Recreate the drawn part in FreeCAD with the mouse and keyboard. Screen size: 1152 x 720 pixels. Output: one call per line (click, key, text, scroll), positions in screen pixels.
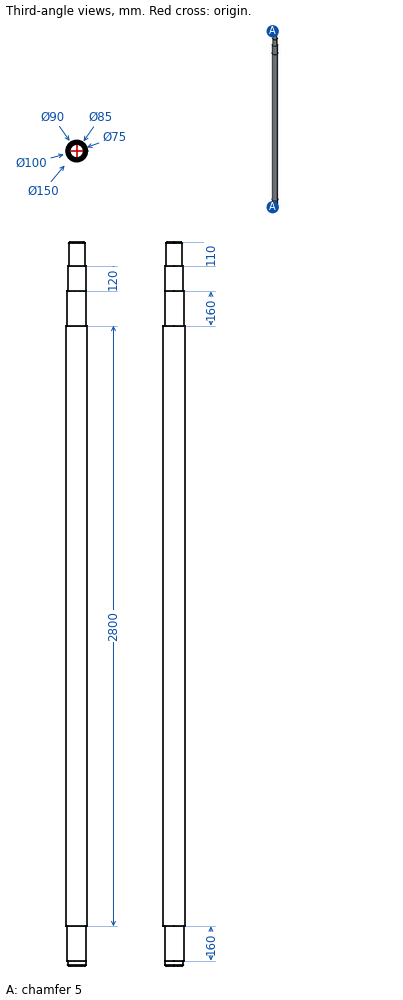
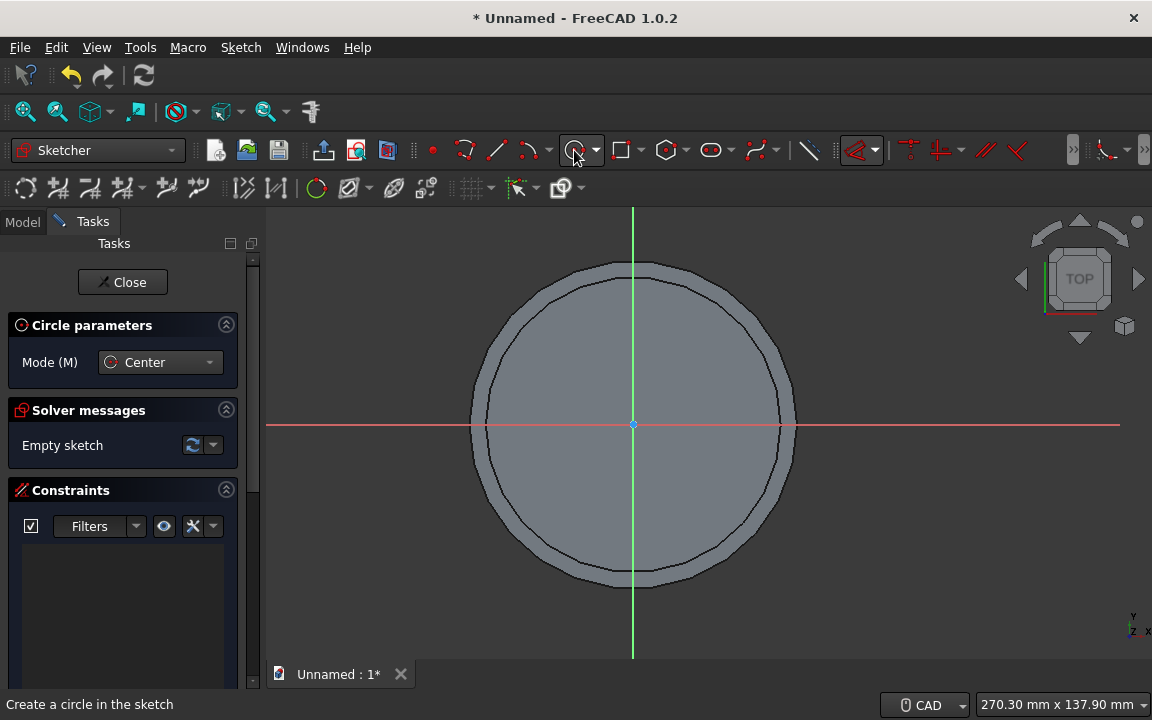
click(633, 425)
click(732, 326)
key(Escape)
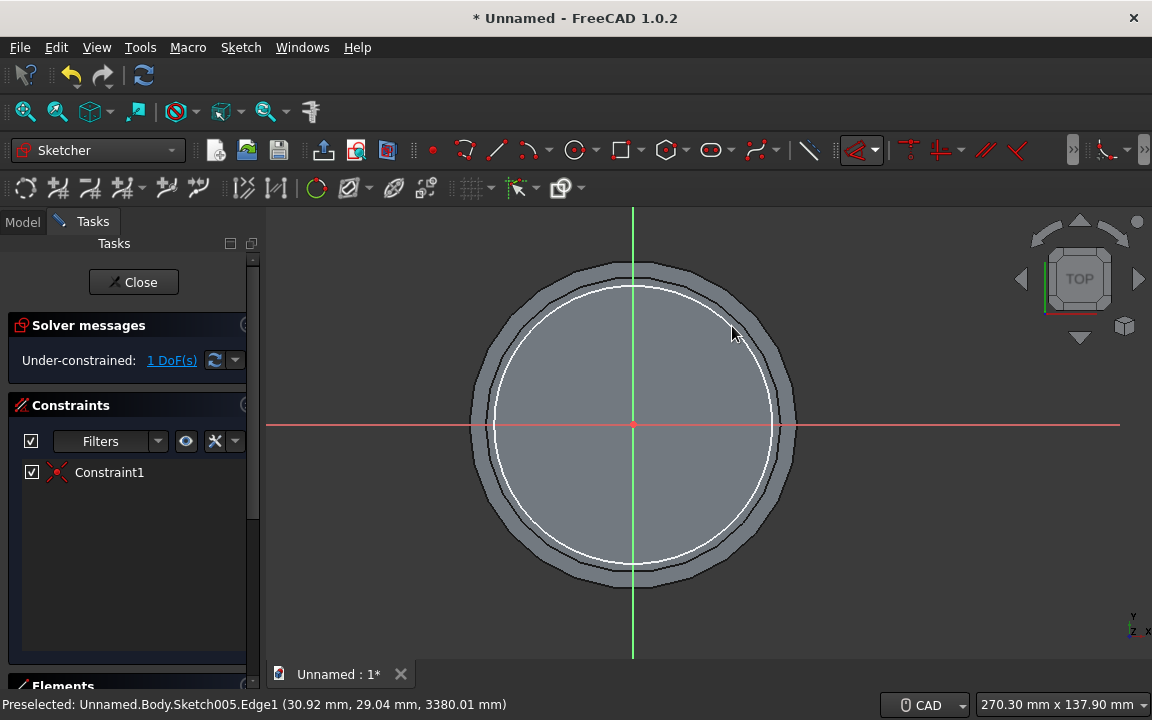
click(731, 326)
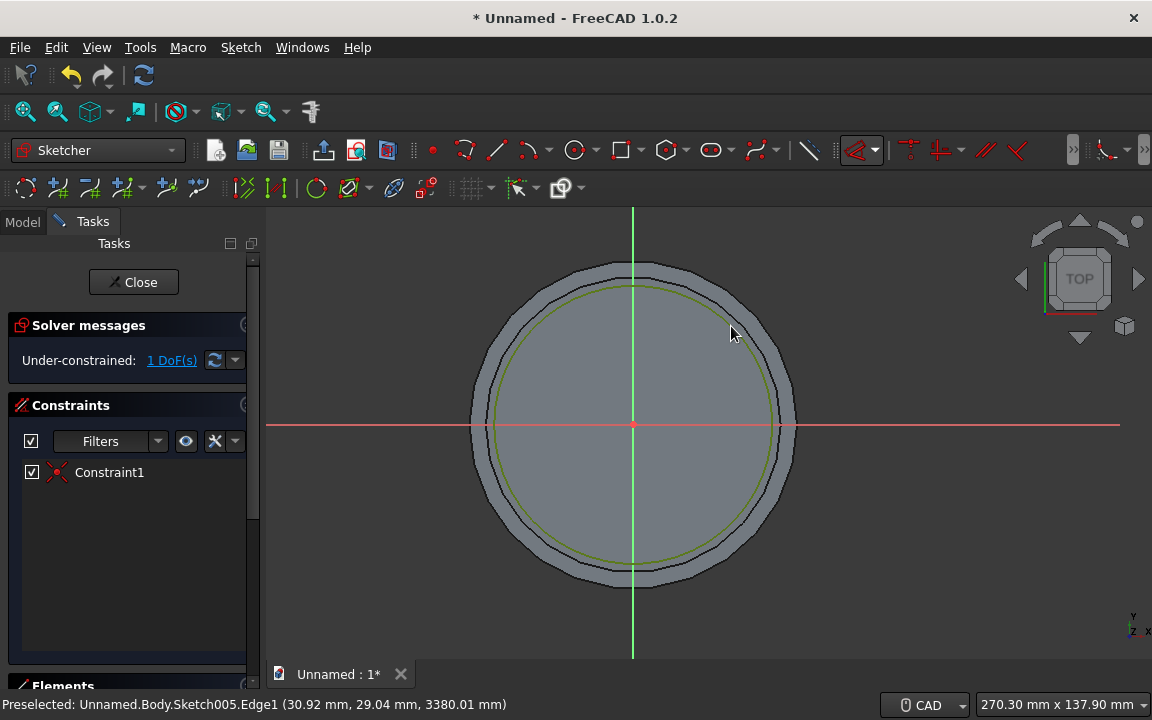
click(878, 150)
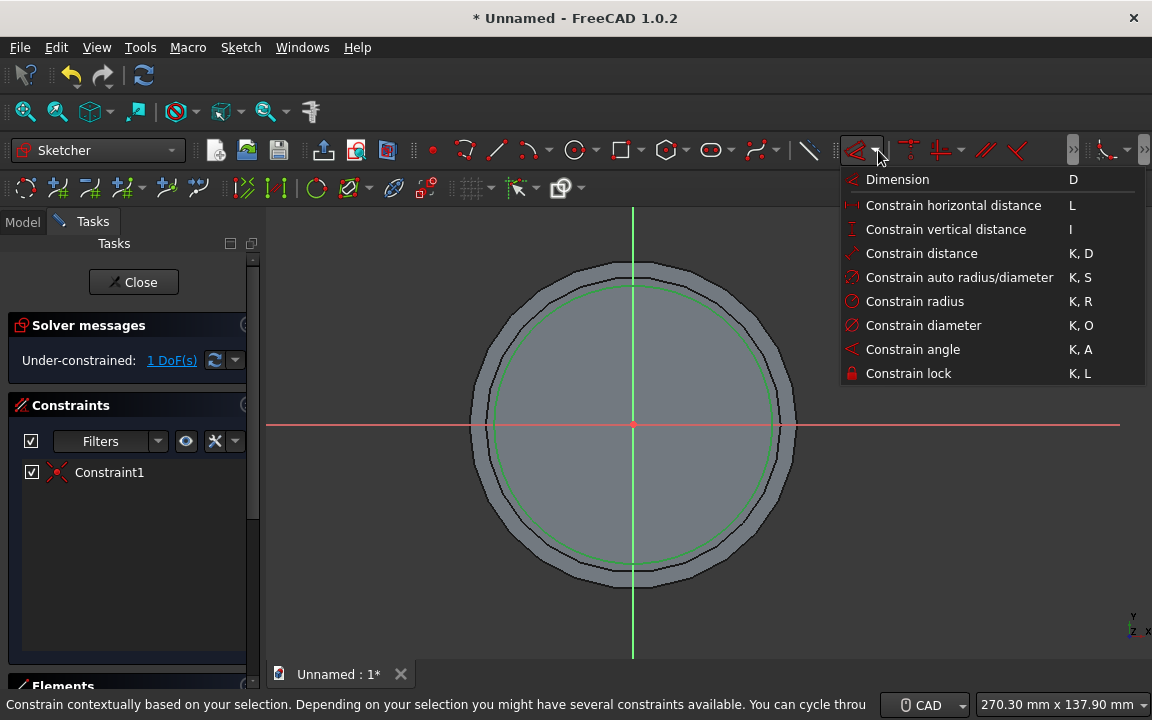
click(993, 325)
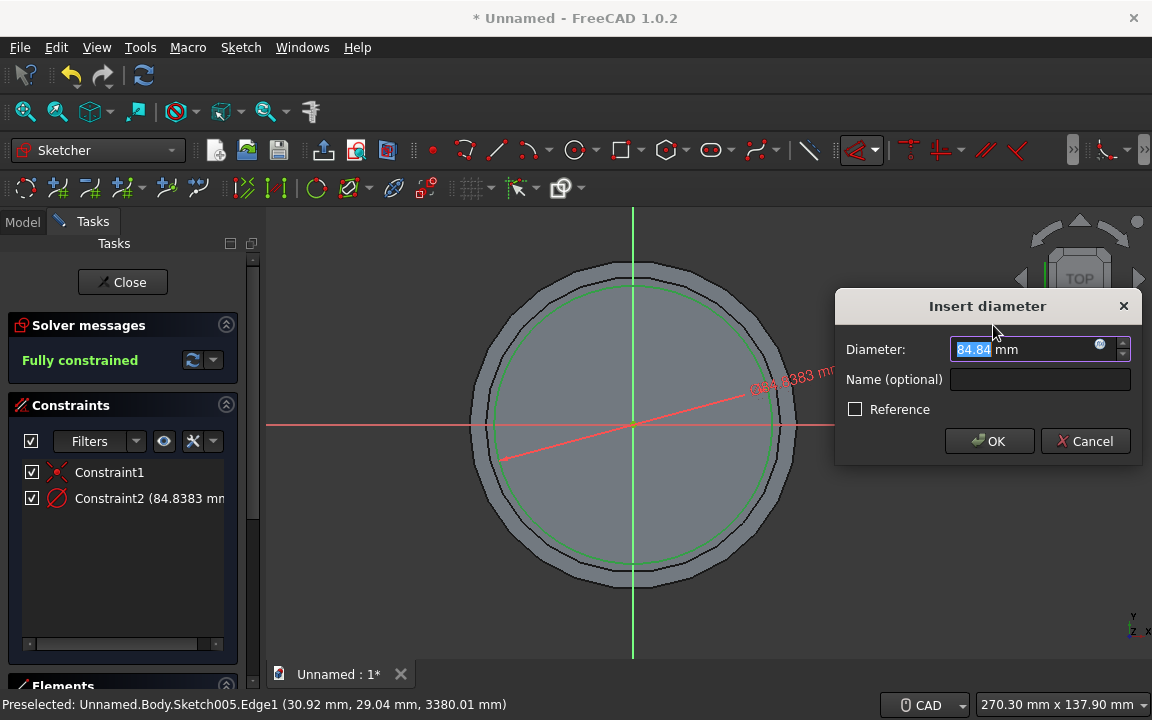
text(85)
key(Return)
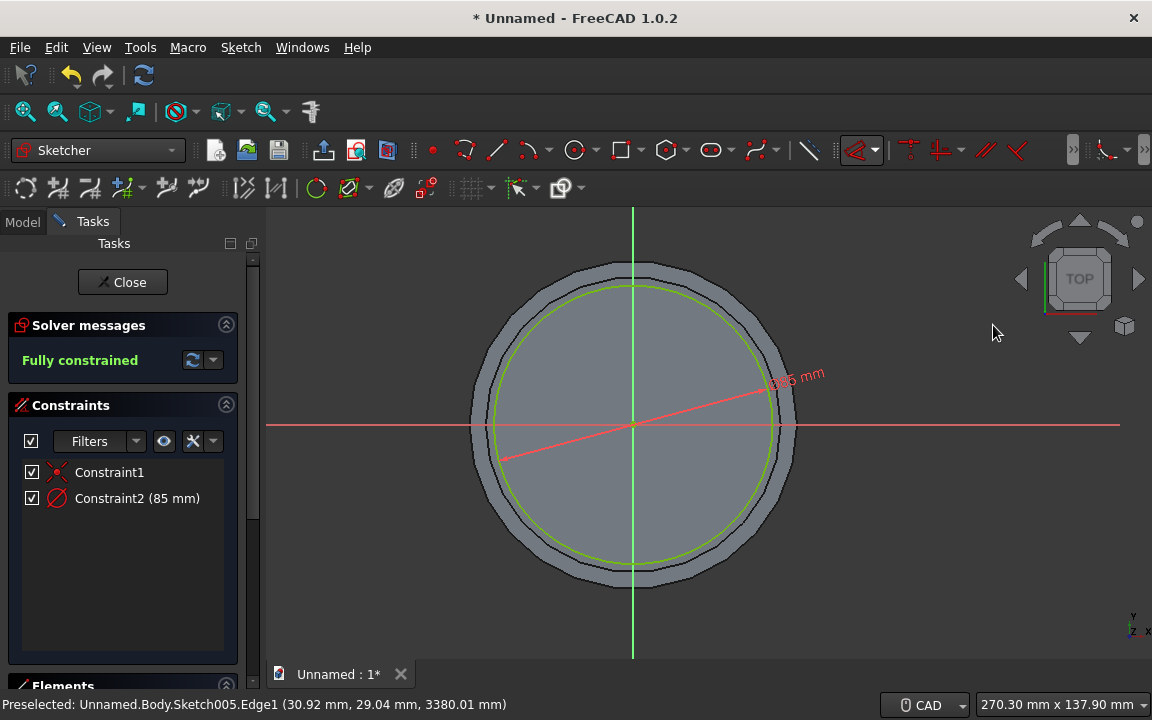
click(123, 282)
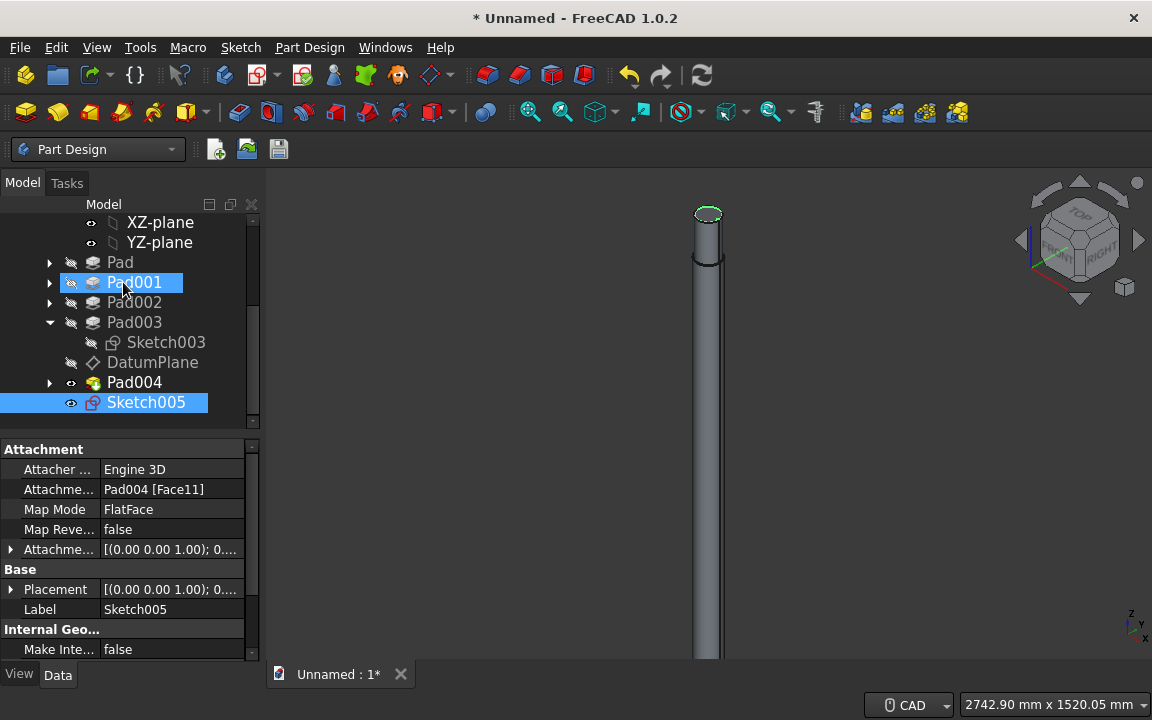
click(26, 112)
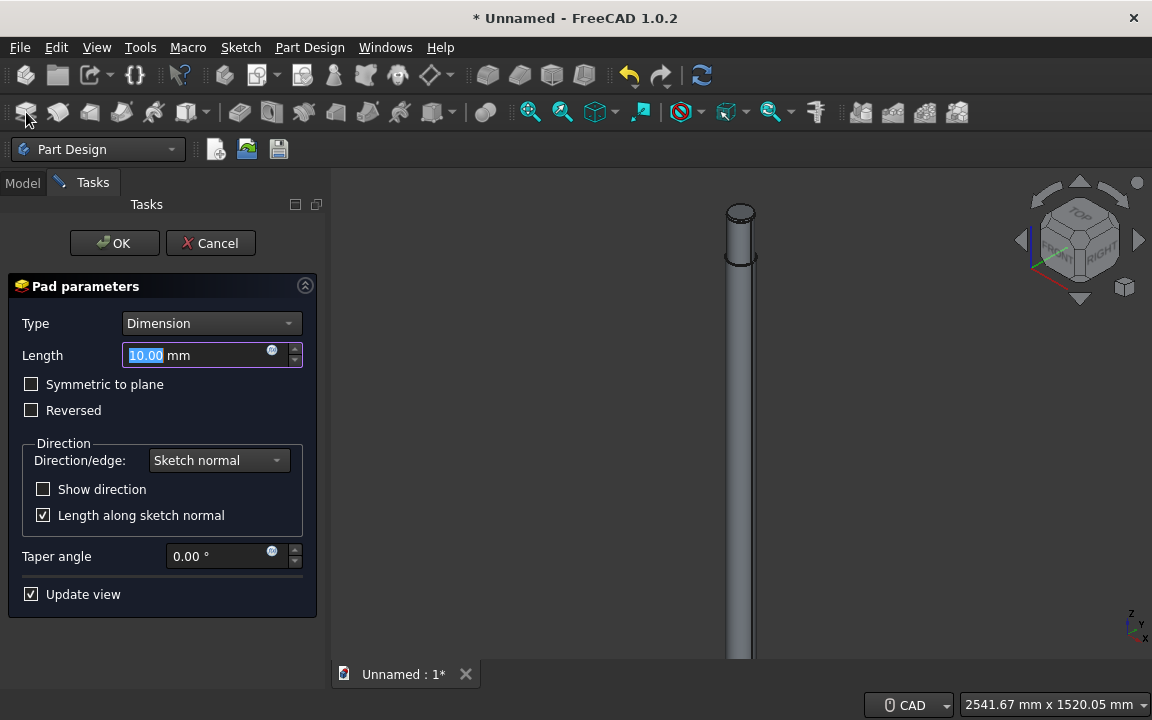
text(120)
key(Tab)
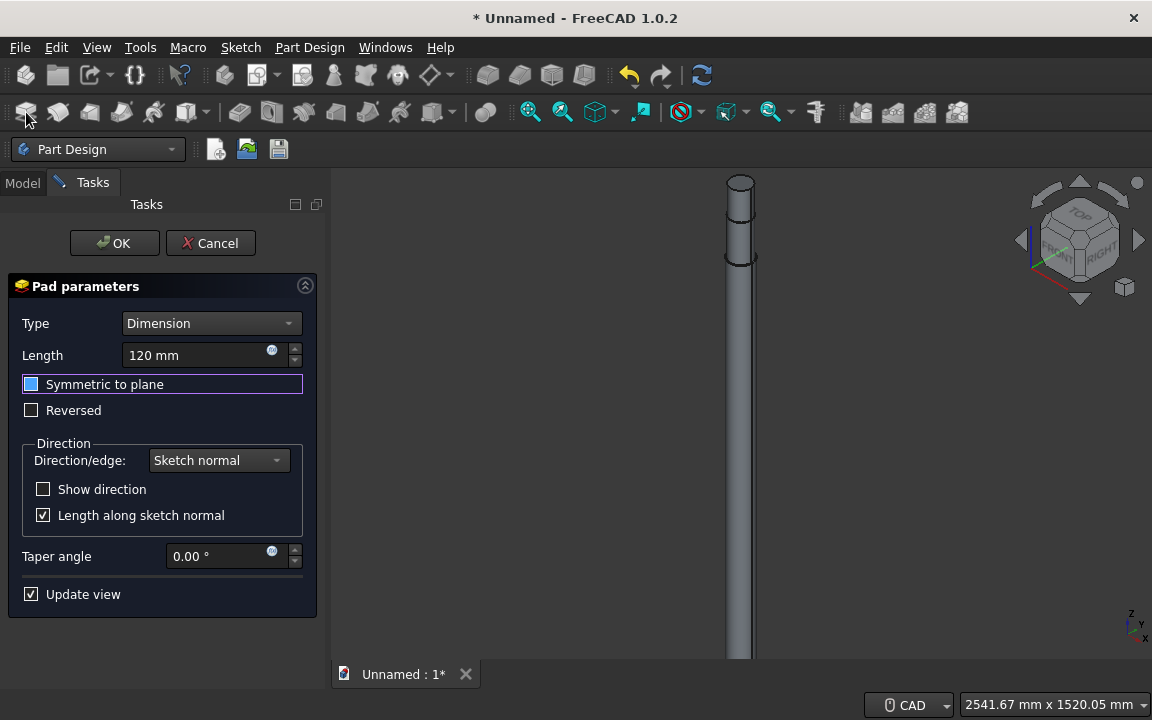
click(115, 243)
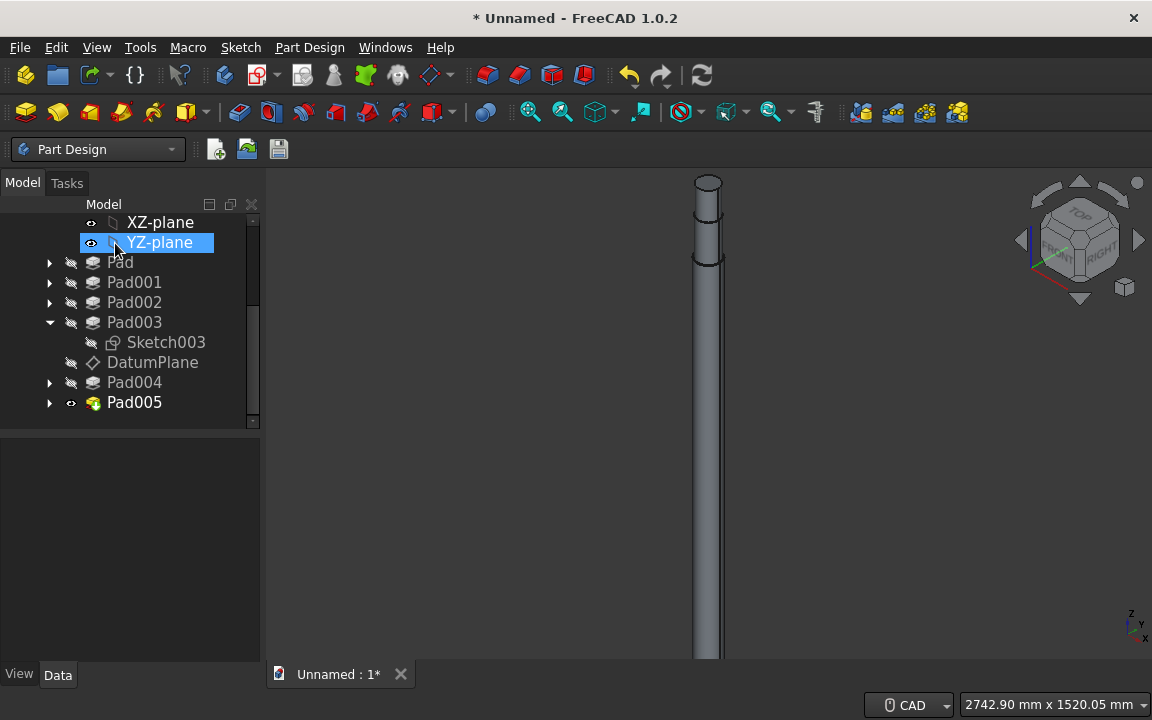
click(532, 112)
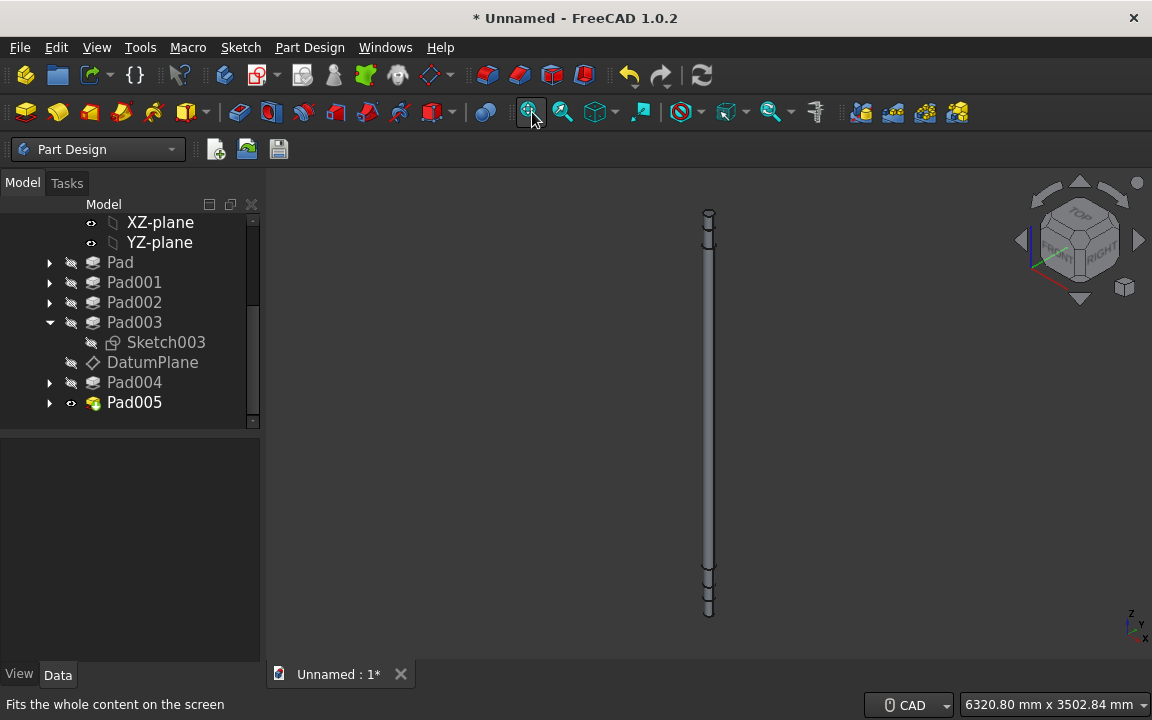
scroll(709, 212, up, 4)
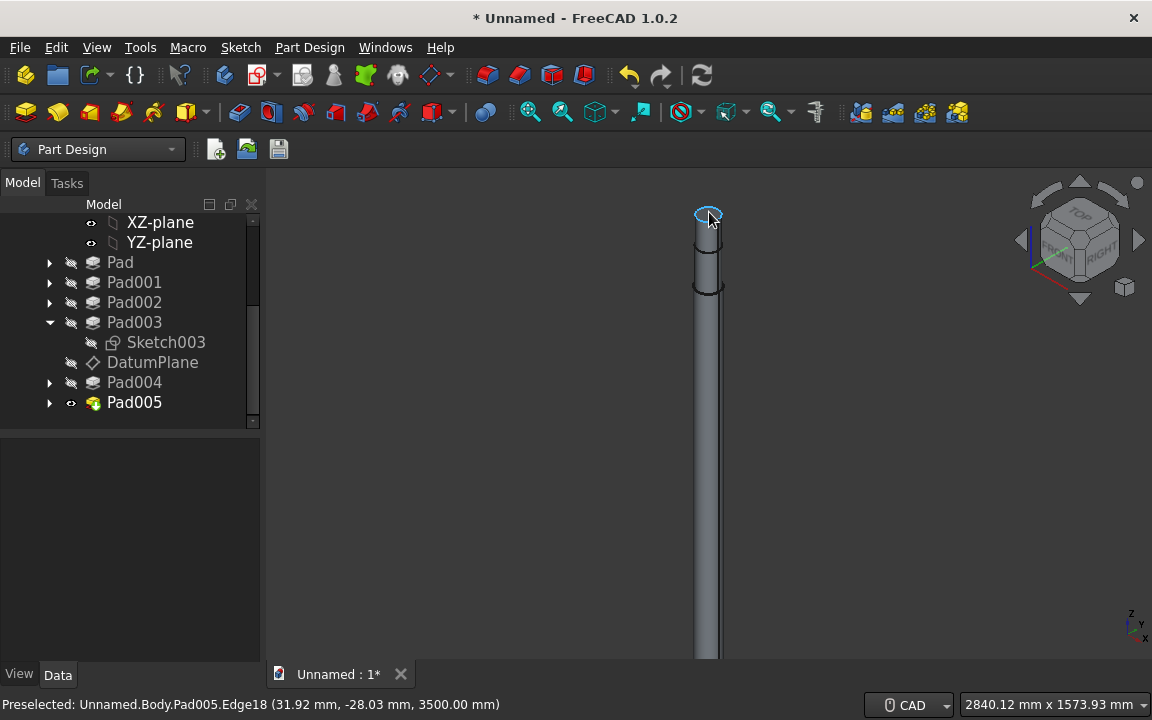
click(711, 212)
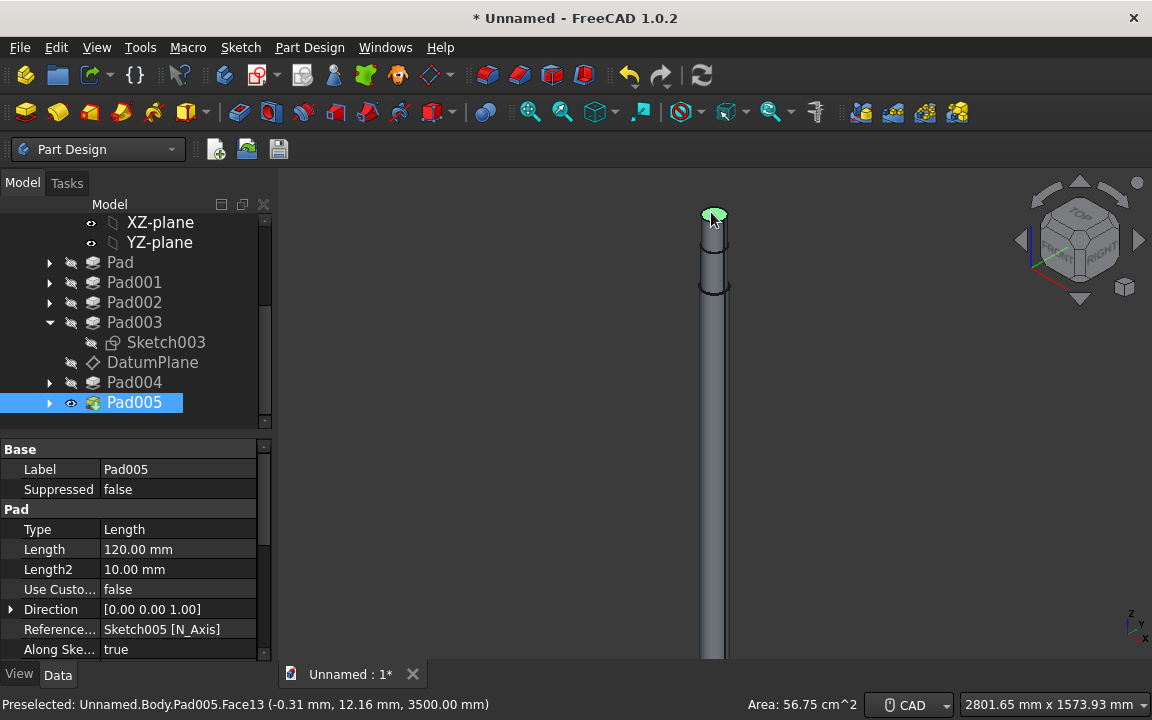
click(258, 76)